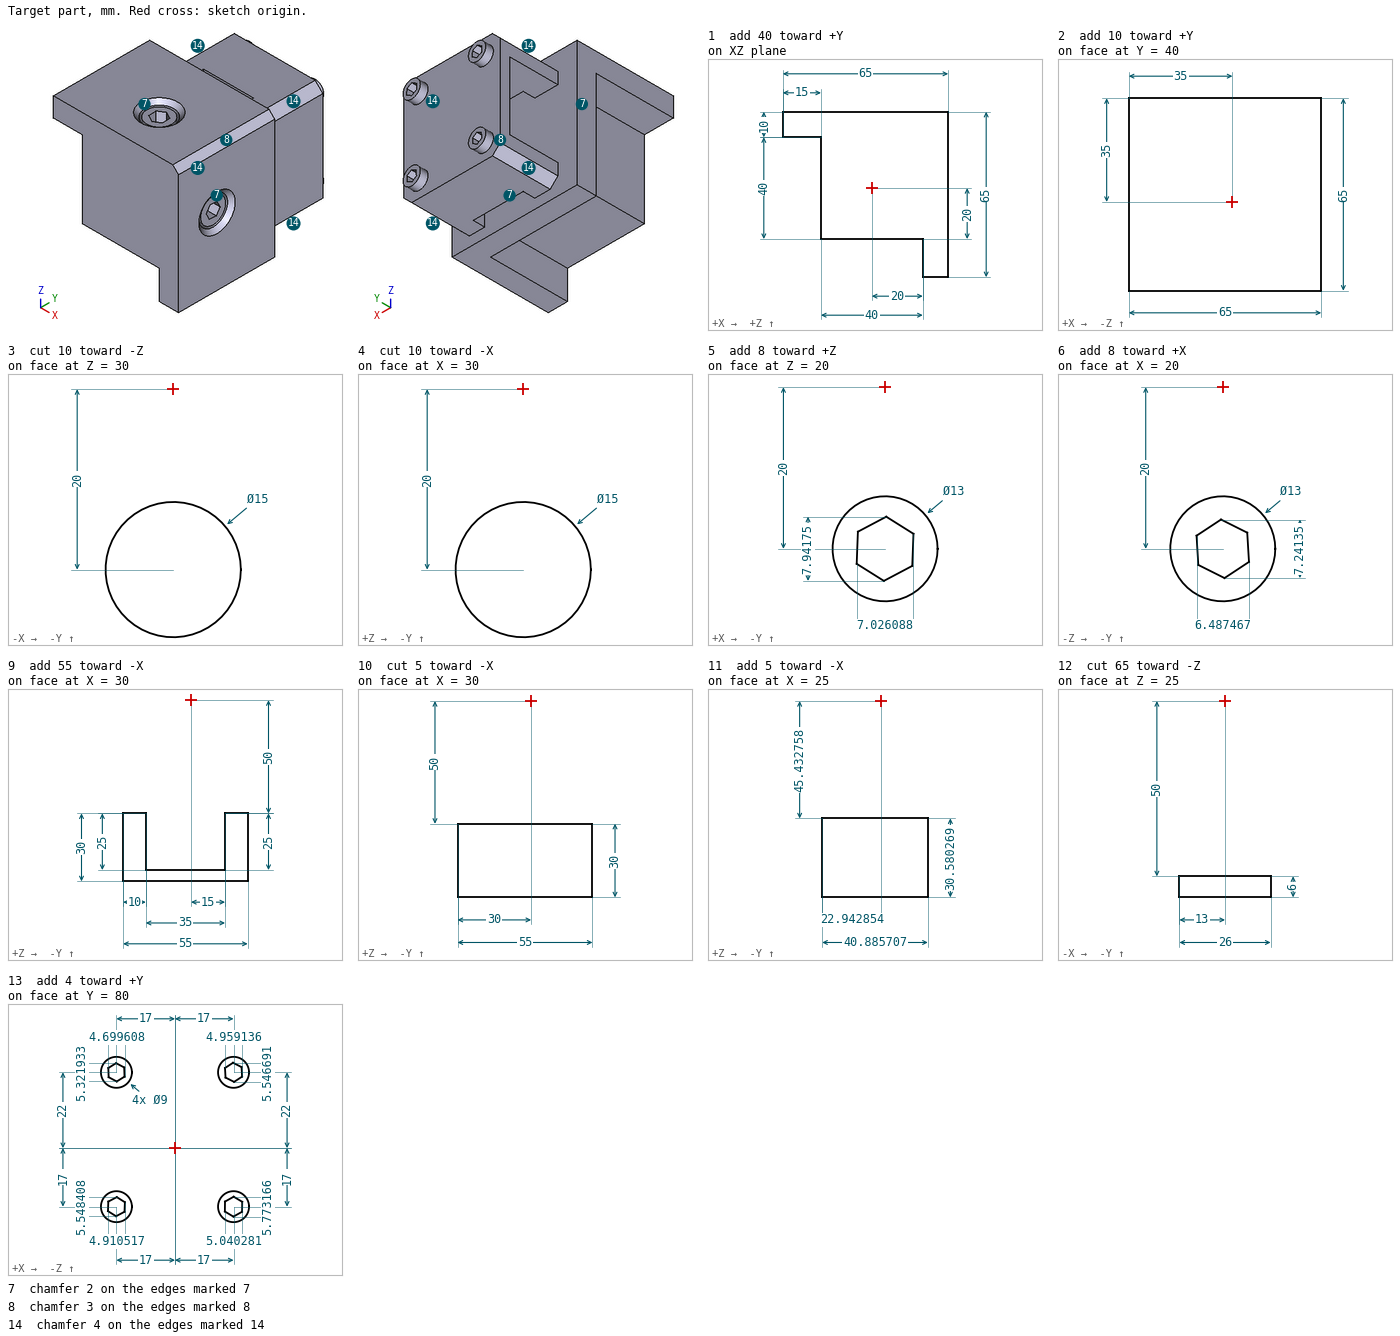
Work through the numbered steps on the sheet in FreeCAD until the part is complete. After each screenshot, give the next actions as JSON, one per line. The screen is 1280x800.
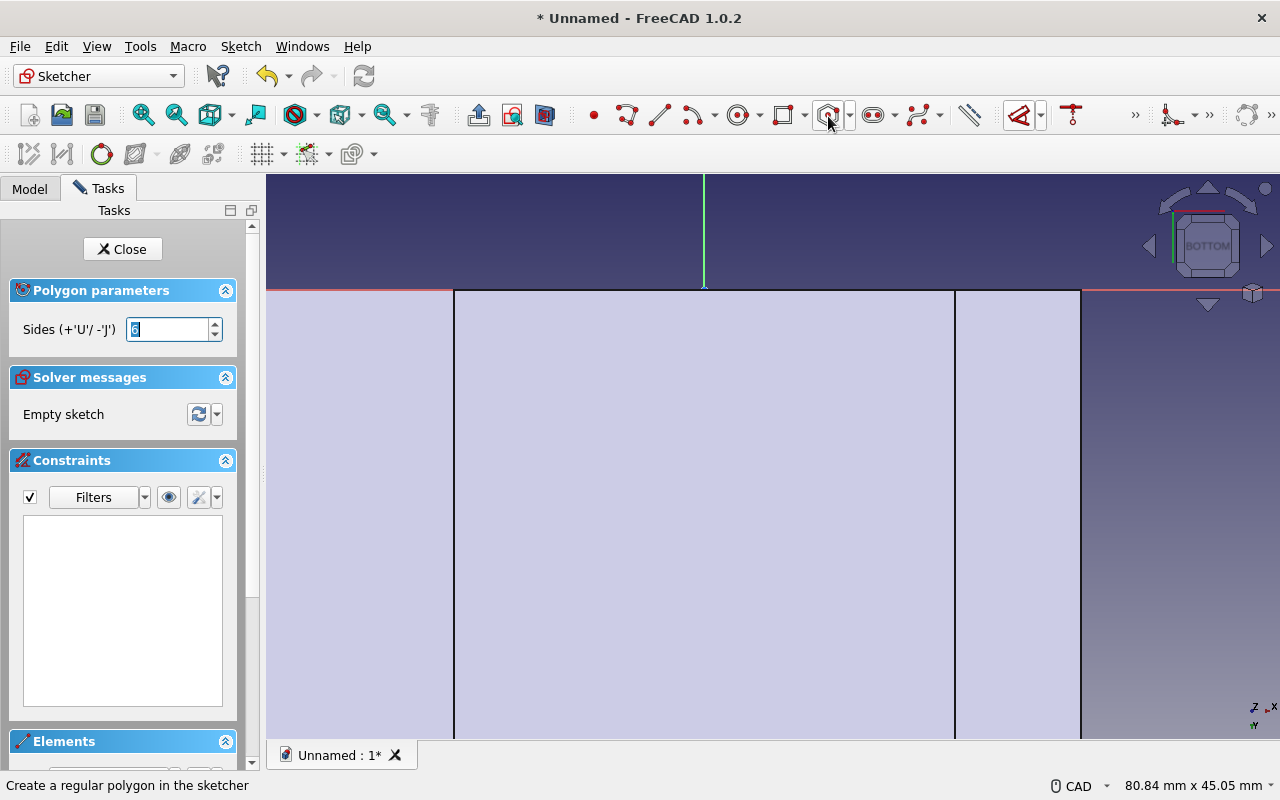
{"action": "left_click", "coordinate": [704, 541]}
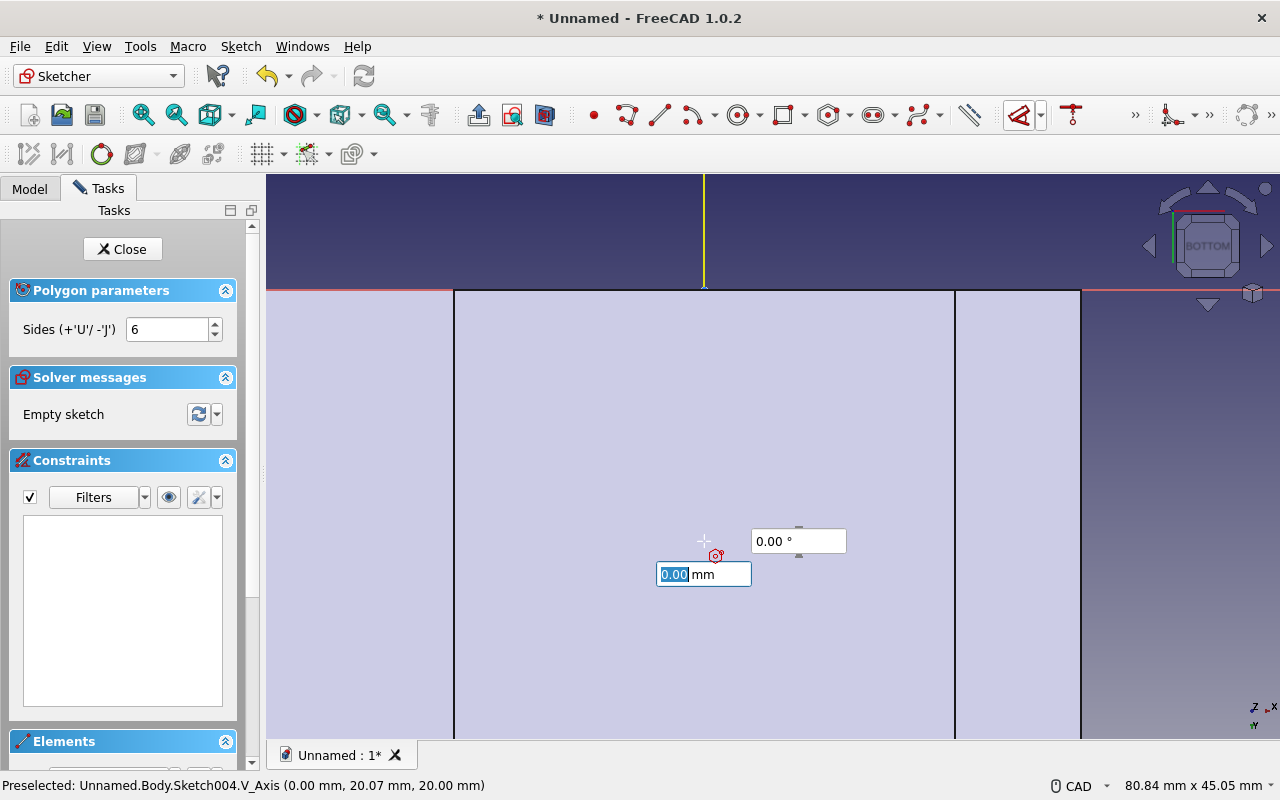
{"action": "left_click", "coordinate": [748, 518]}
{"action": "right_click", "coordinate": [748, 518]}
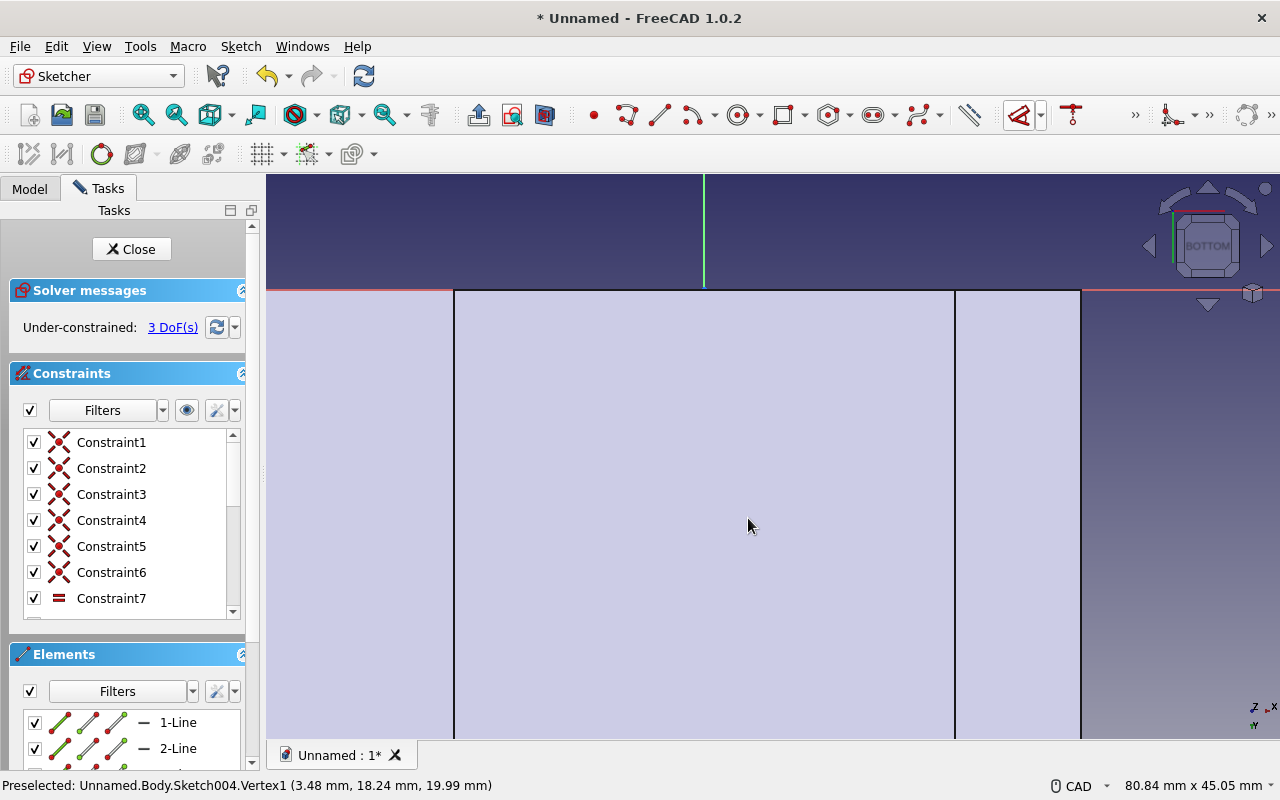
{"action": "left_click", "coordinate": [738, 116]}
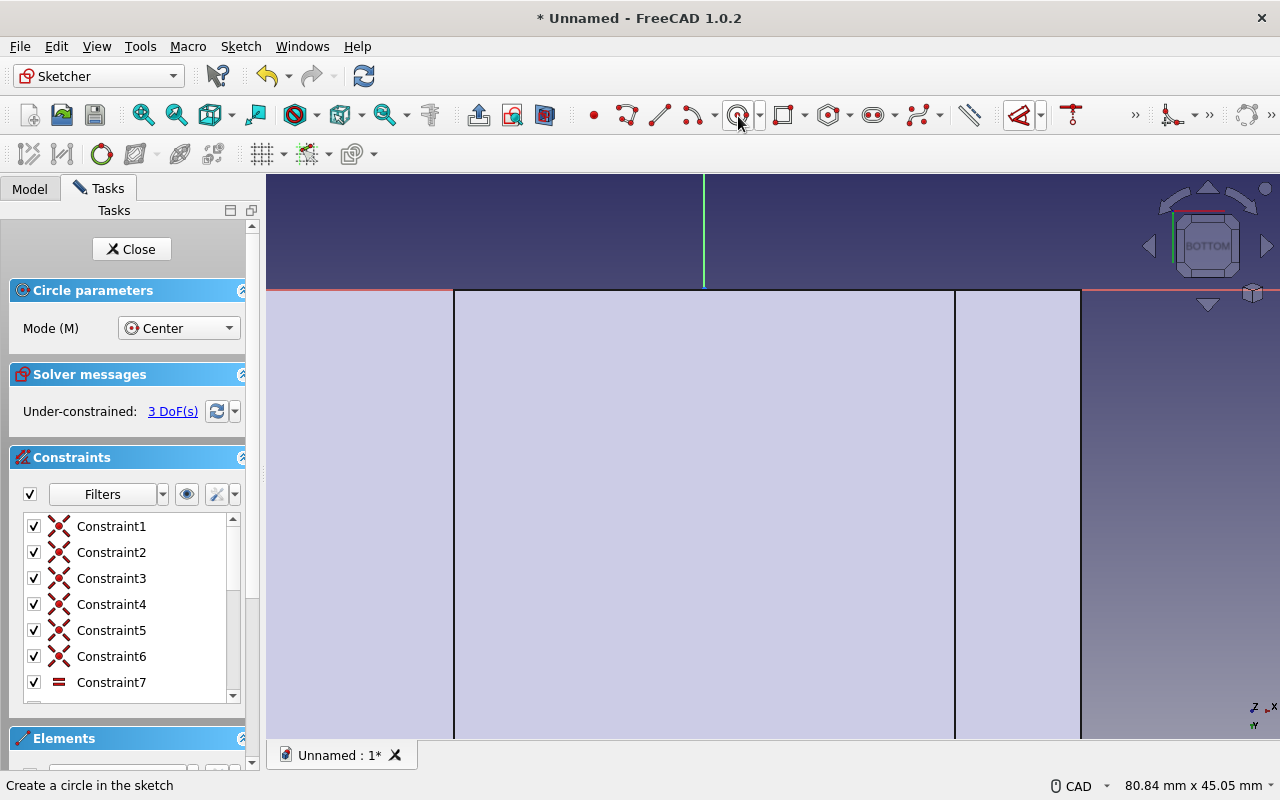
{"action": "left_click", "coordinate": [704, 542]}
{"action": "mouse_move", "coordinate": [762, 483]}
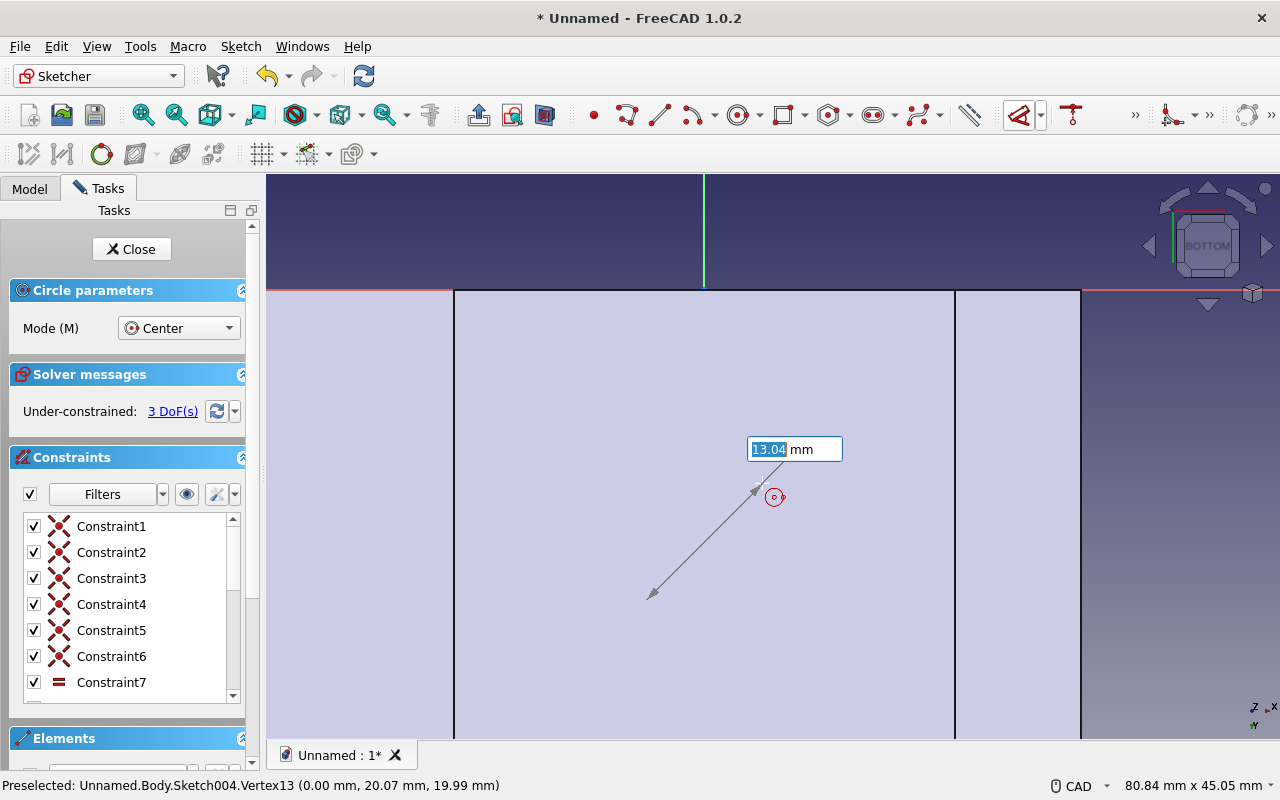
{"action": "type", "text": "13"}
{"action": "key", "text": "Return"}
{"action": "key", "text": "Escape"}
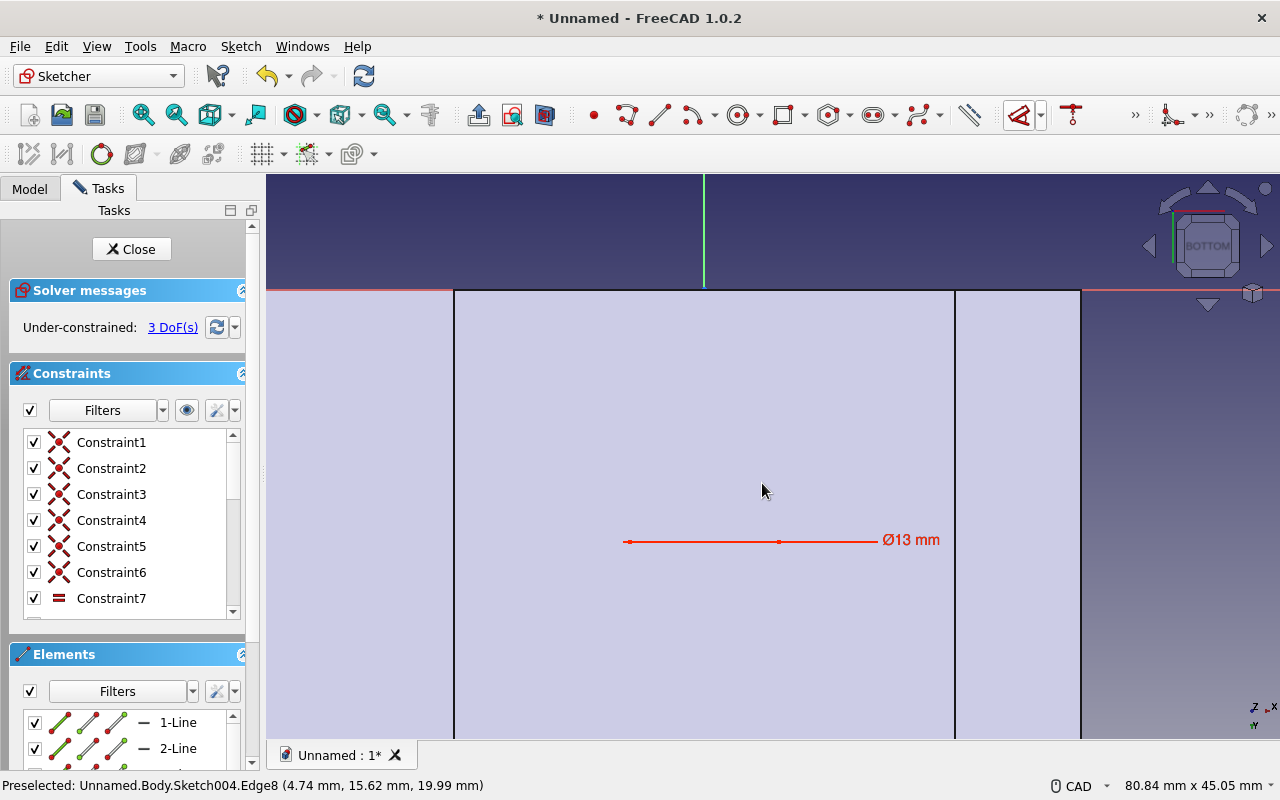
{"action": "left_click", "coordinate": [704, 542]}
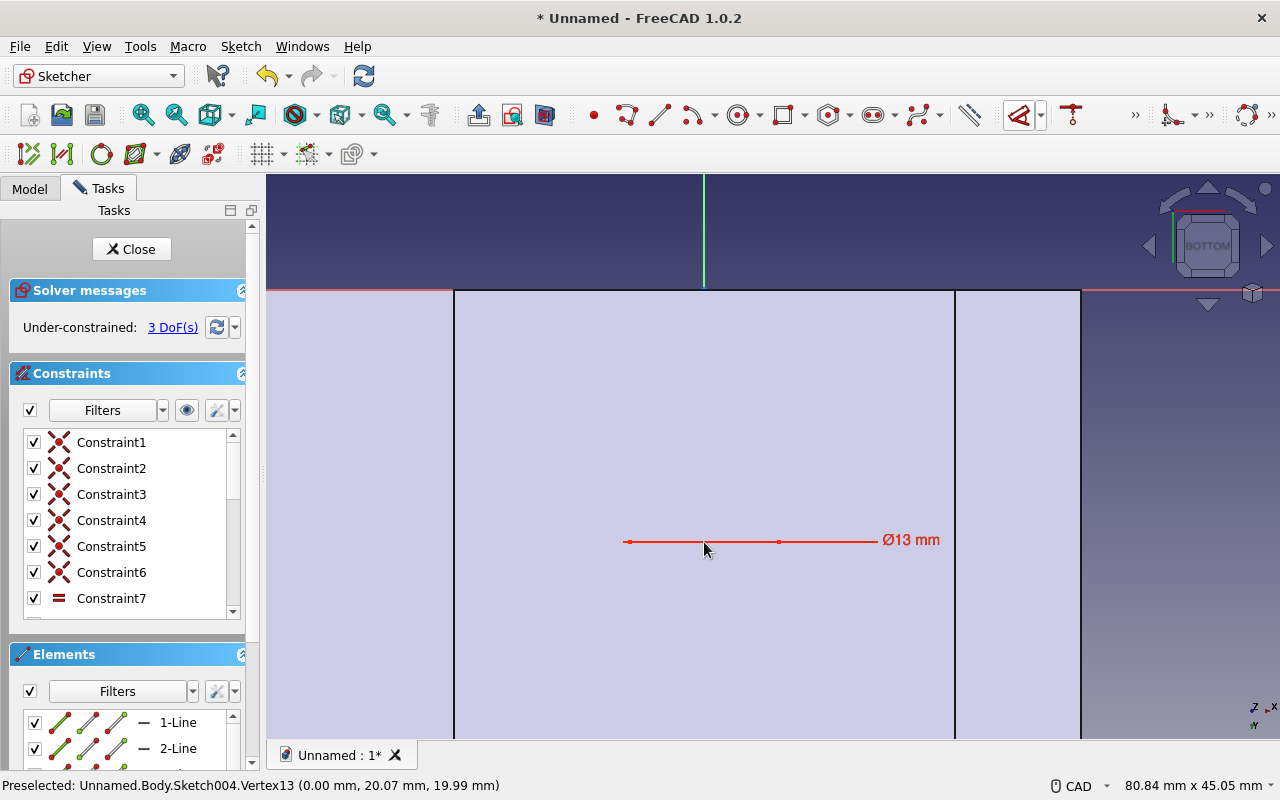
{"action": "left_click", "coordinate": [1040, 116]}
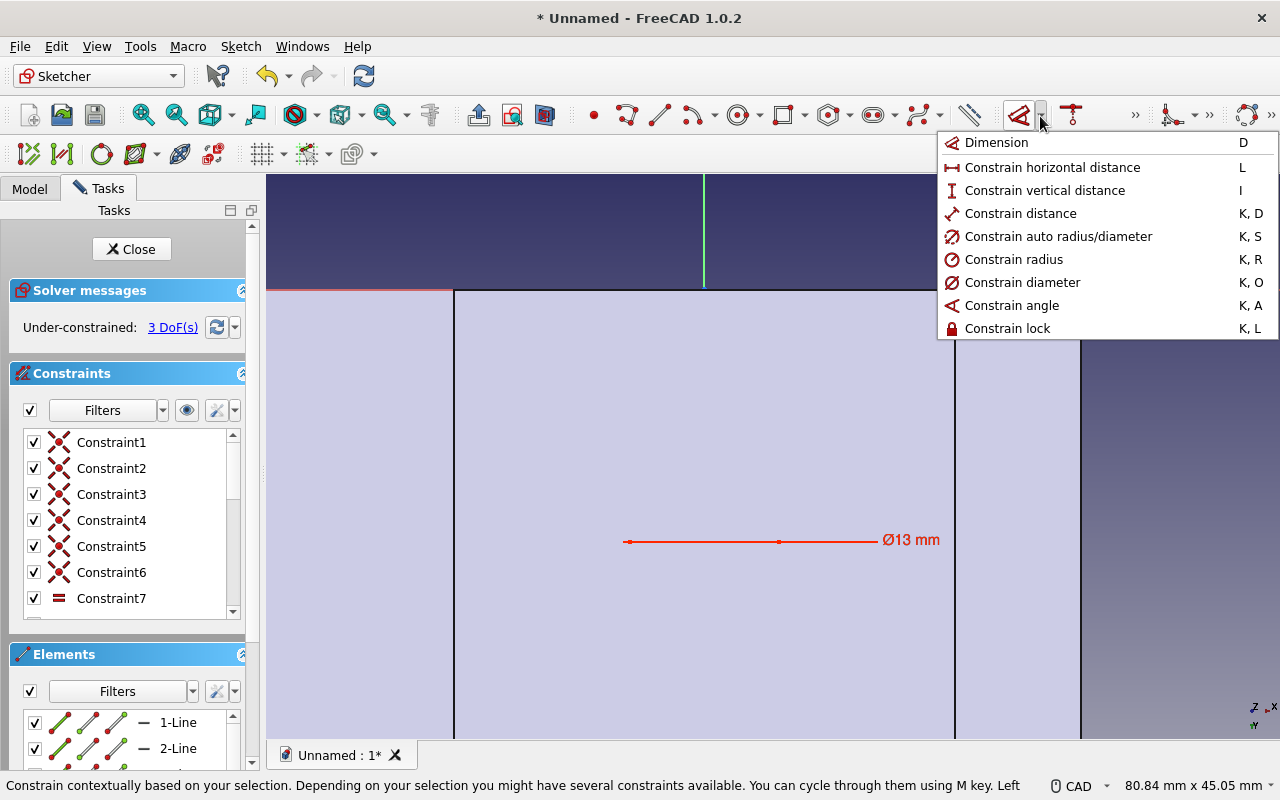
{"action": "left_click", "coordinate": [1108, 190]}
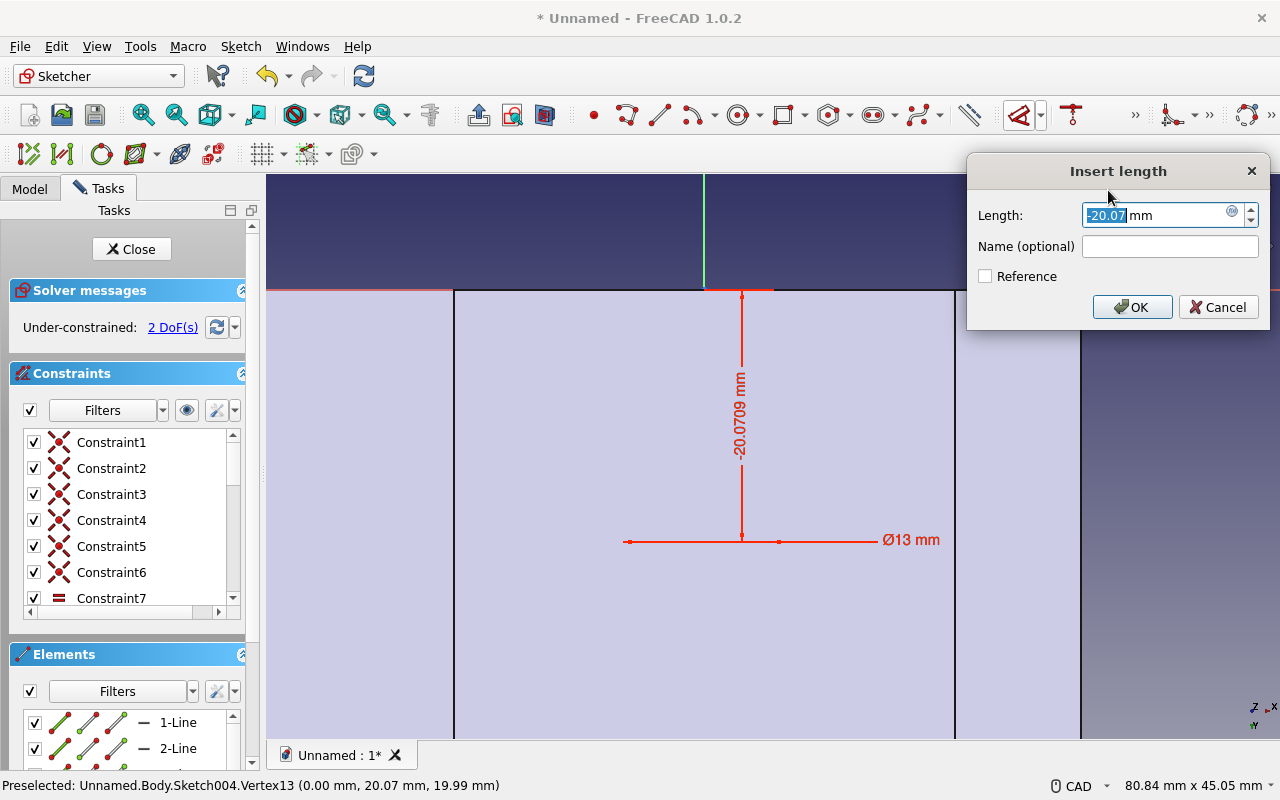
{"action": "type", "text": "-20"}
{"action": "key", "text": "Return"}